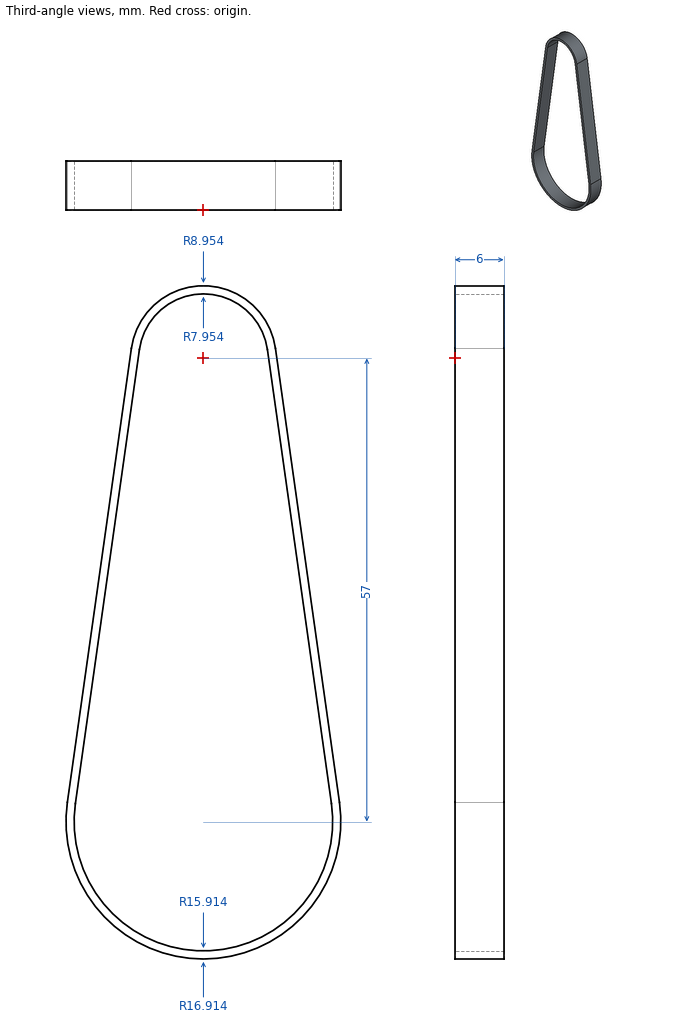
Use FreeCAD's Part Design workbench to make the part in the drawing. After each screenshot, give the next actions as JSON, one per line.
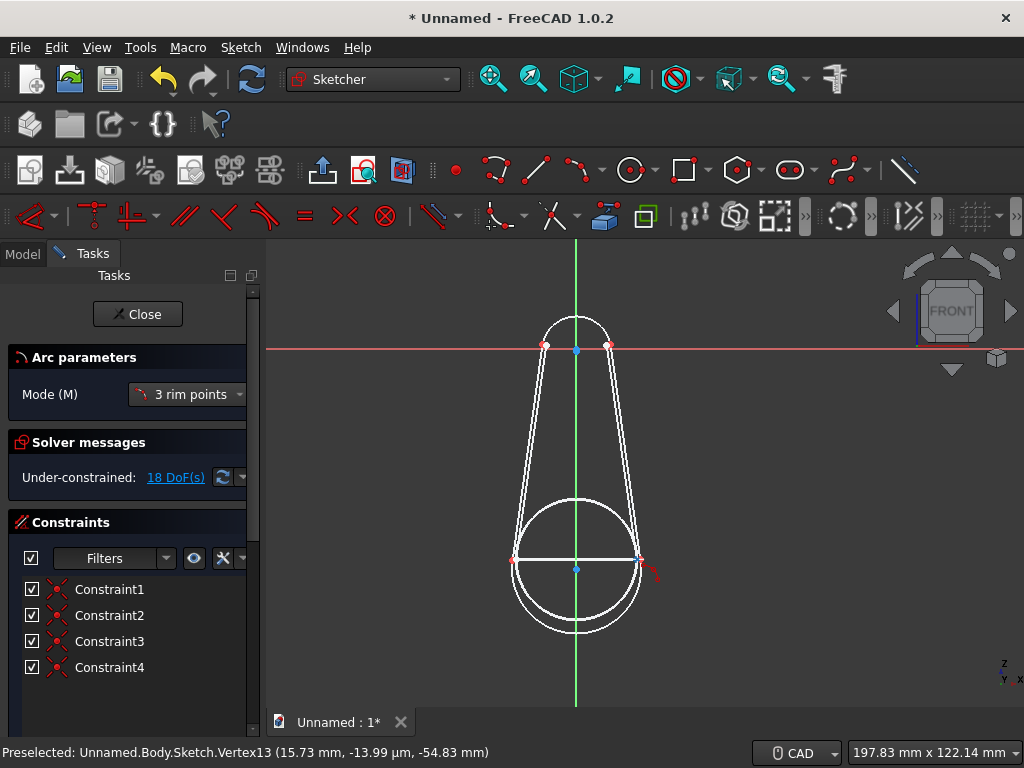
{"action": "scroll", "coordinate": [615, 615], "scroll_direction": "up", "scroll_amount": 8}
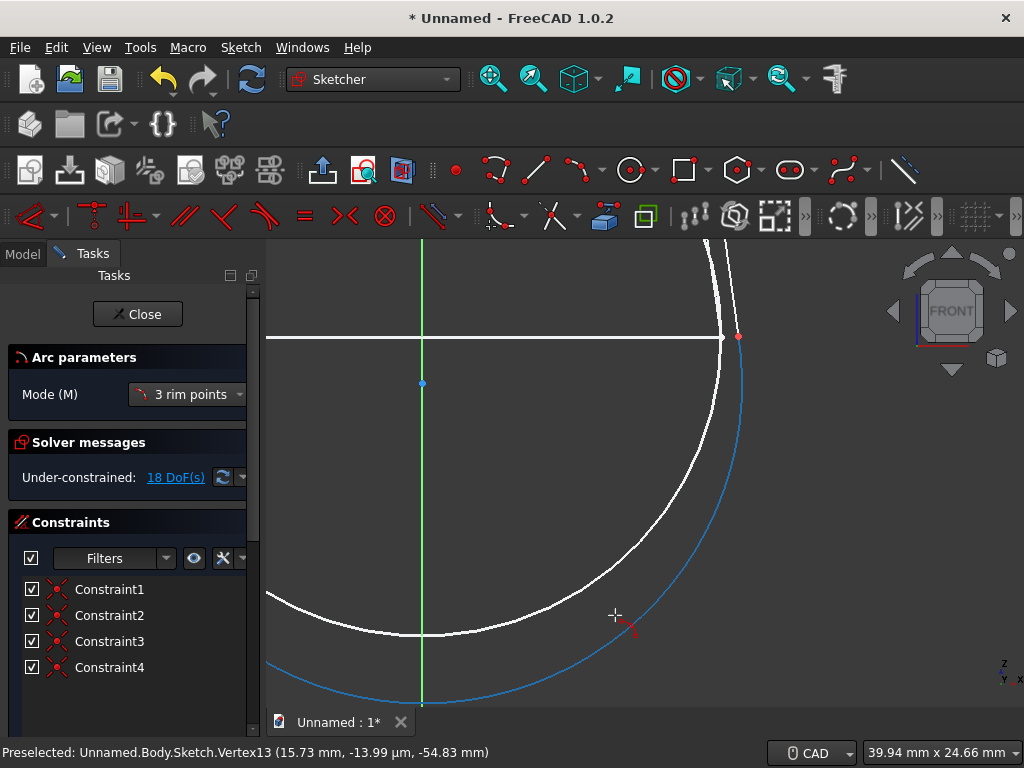
{"action": "left_click", "coordinate": [613, 612]}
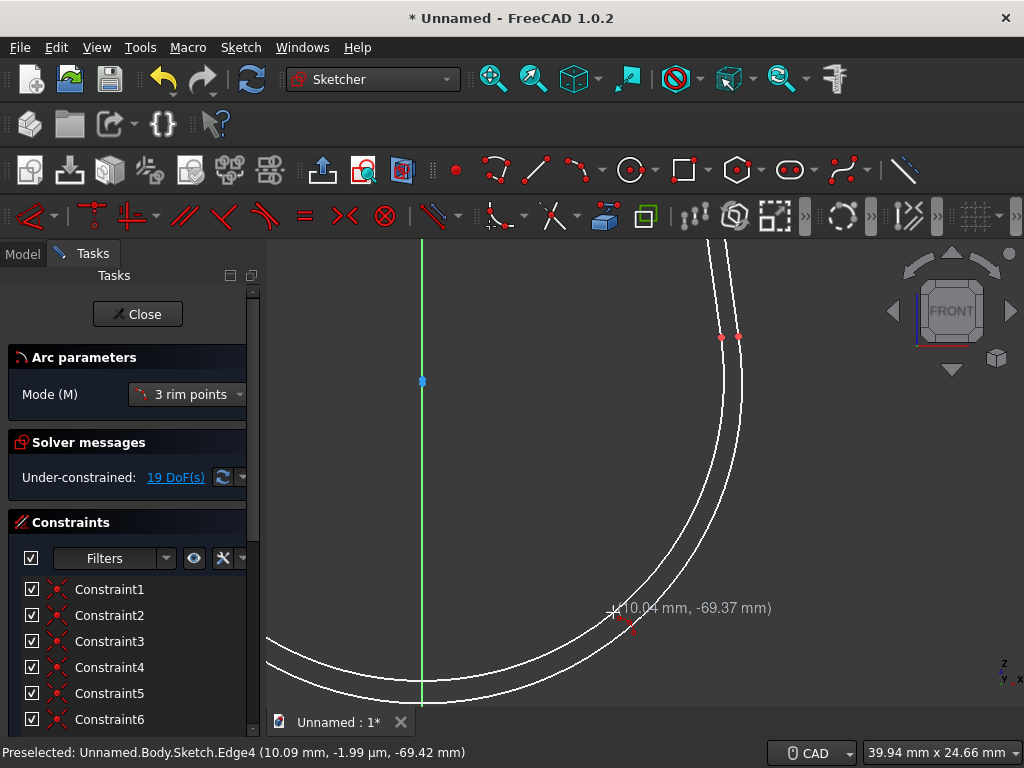
{"action": "scroll", "coordinate": [615, 615], "scroll_direction": "down", "scroll_amount": 8}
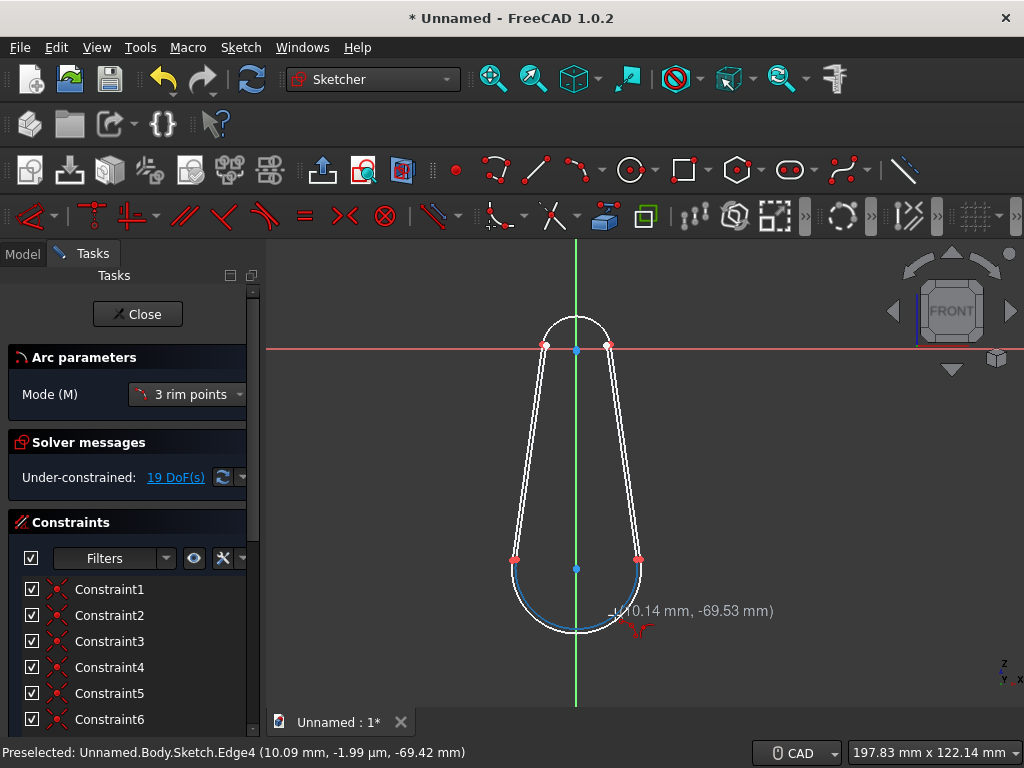
{"action": "scroll", "coordinate": [607, 345], "scroll_direction": "up", "scroll_amount": 8}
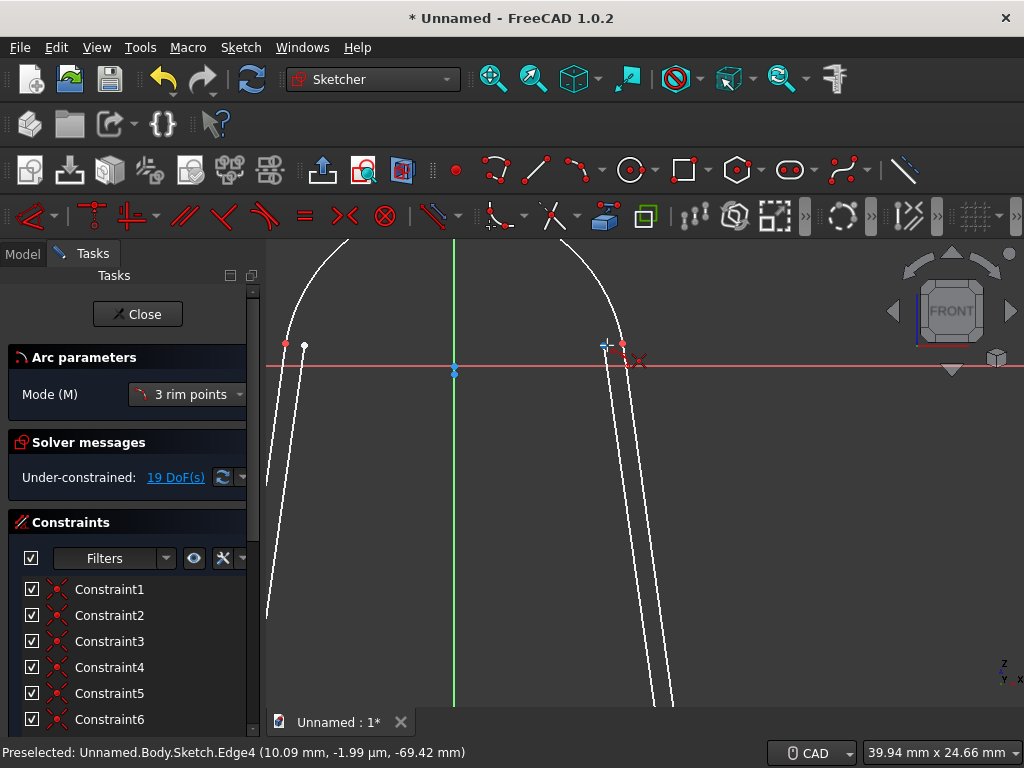
{"action": "left_click", "coordinate": [604, 346]}
{"action": "left_click", "coordinate": [305, 346]}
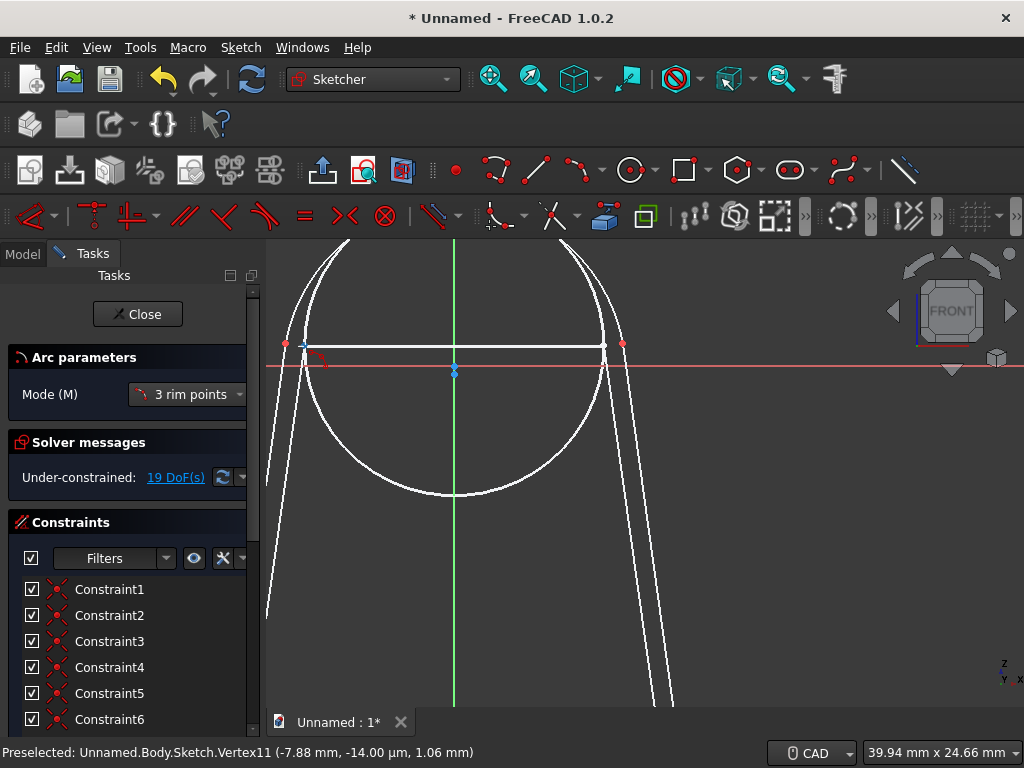
{"action": "scroll", "coordinate": [607, 344], "scroll_direction": "down", "scroll_amount": 8}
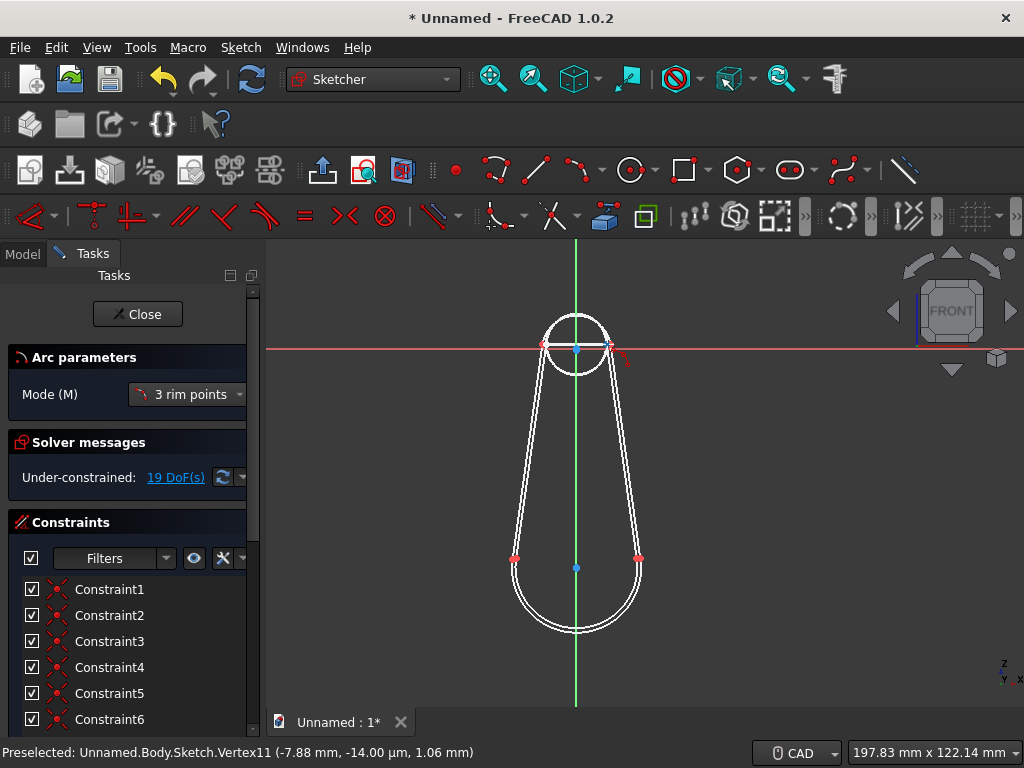
{"action": "scroll", "coordinate": [585, 319], "scroll_direction": "up", "scroll_amount": 8}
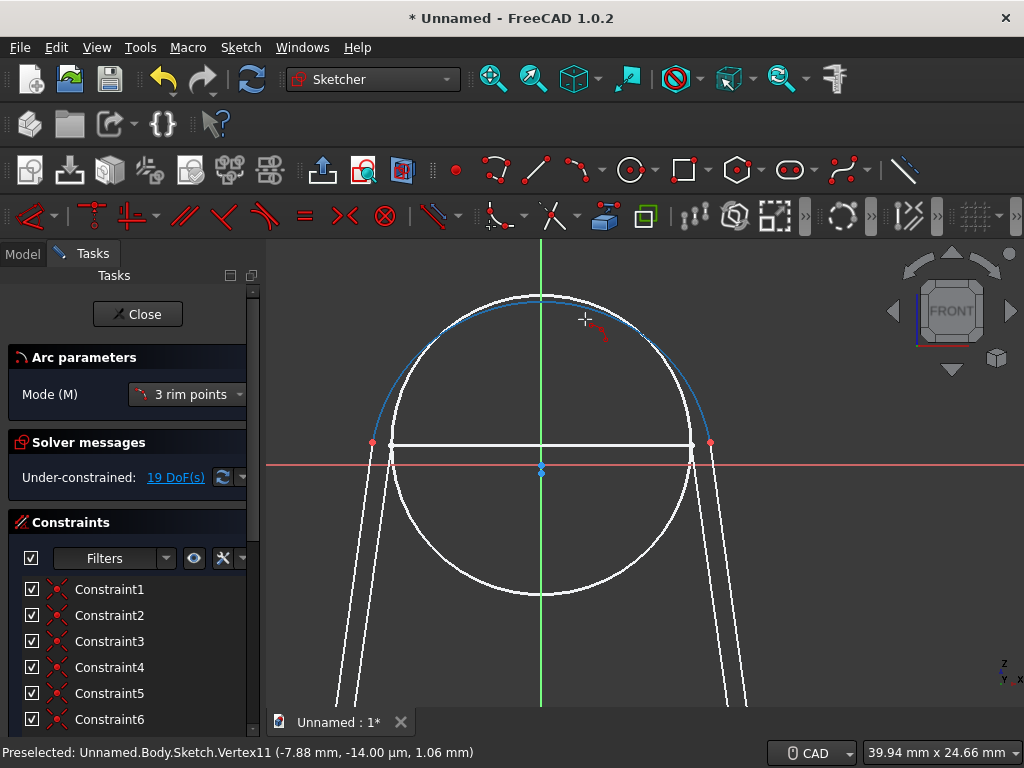
{"action": "left_click", "coordinate": [584, 320]}
{"action": "key", "text": "Escape"}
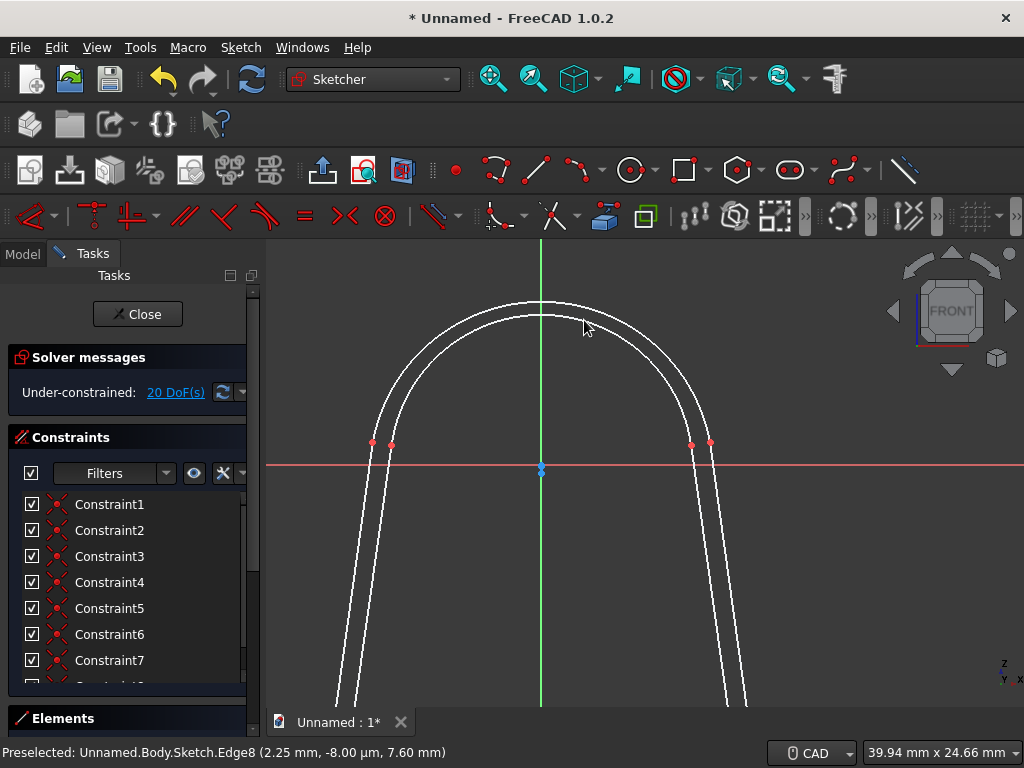
{"action": "left_click", "coordinate": [343, 656]}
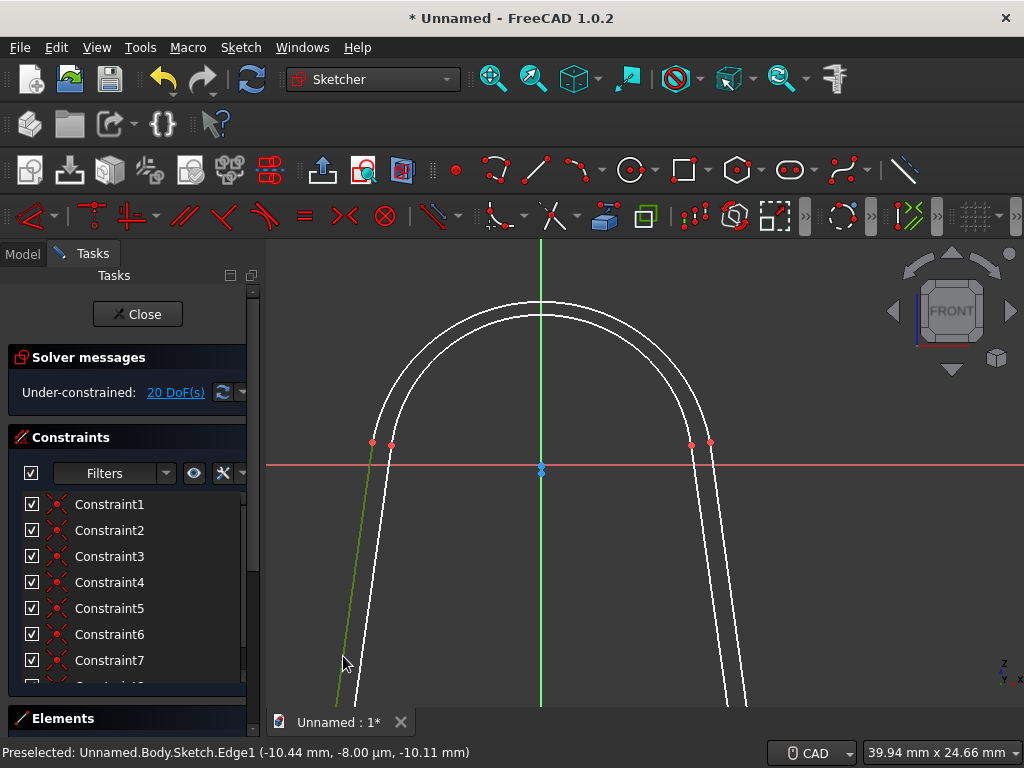
{"action": "left_click", "coordinate": [632, 328]}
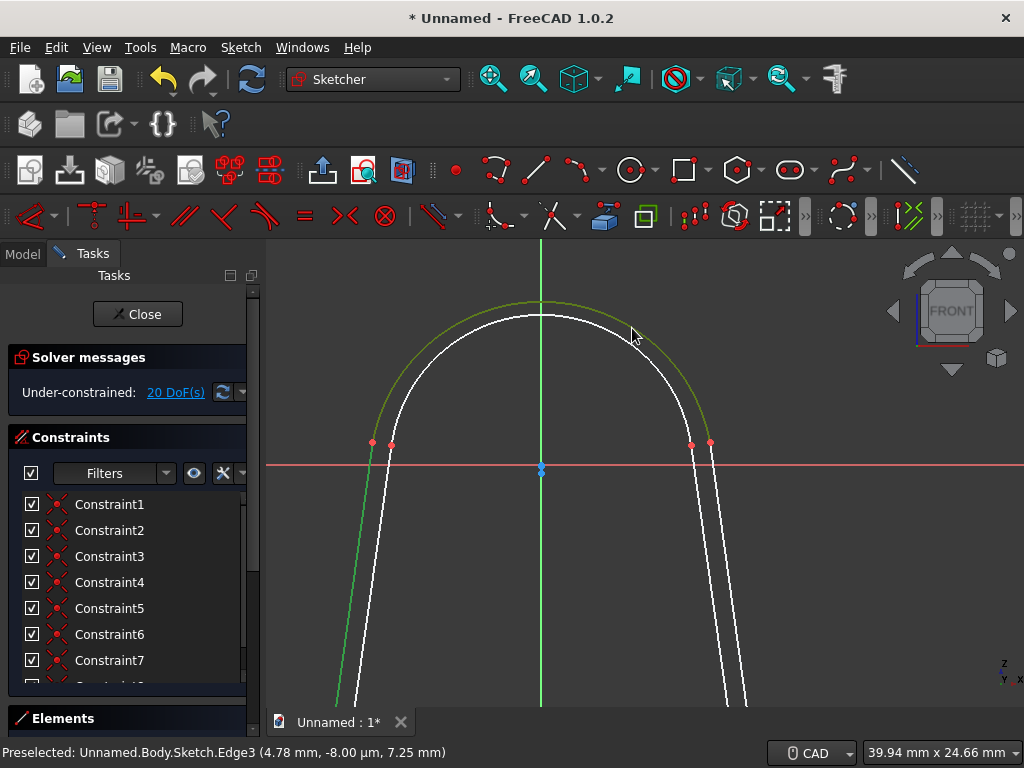
{"action": "left_click", "coordinate": [266, 216]}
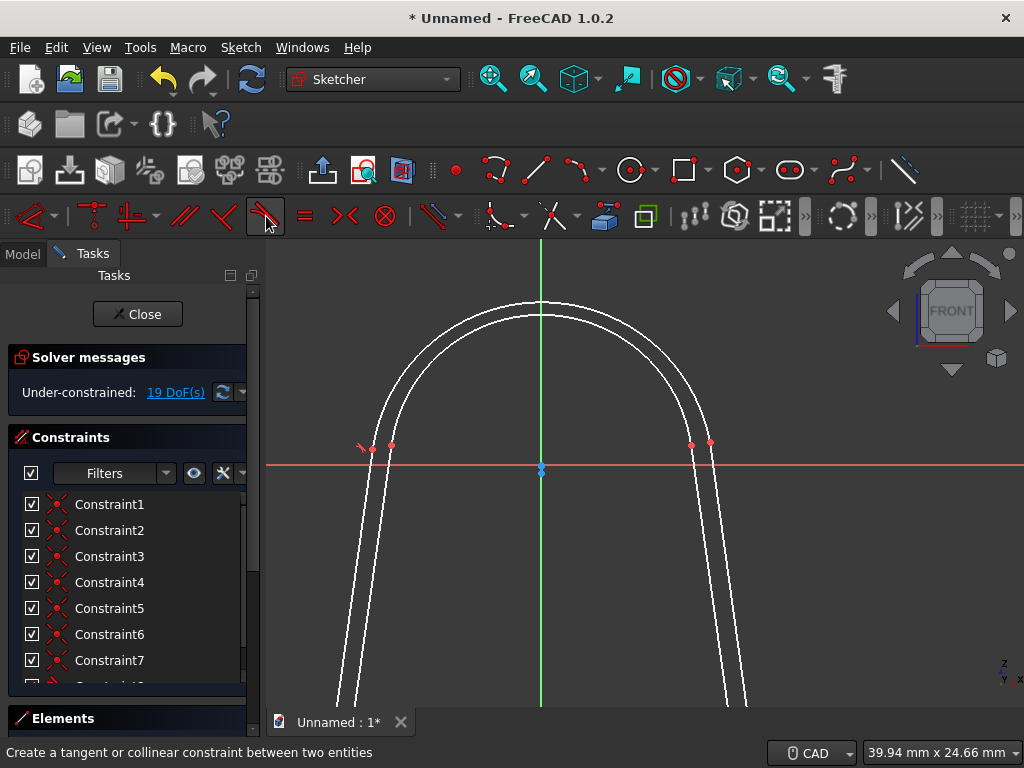
{"action": "left_click", "coordinate": [343, 661]}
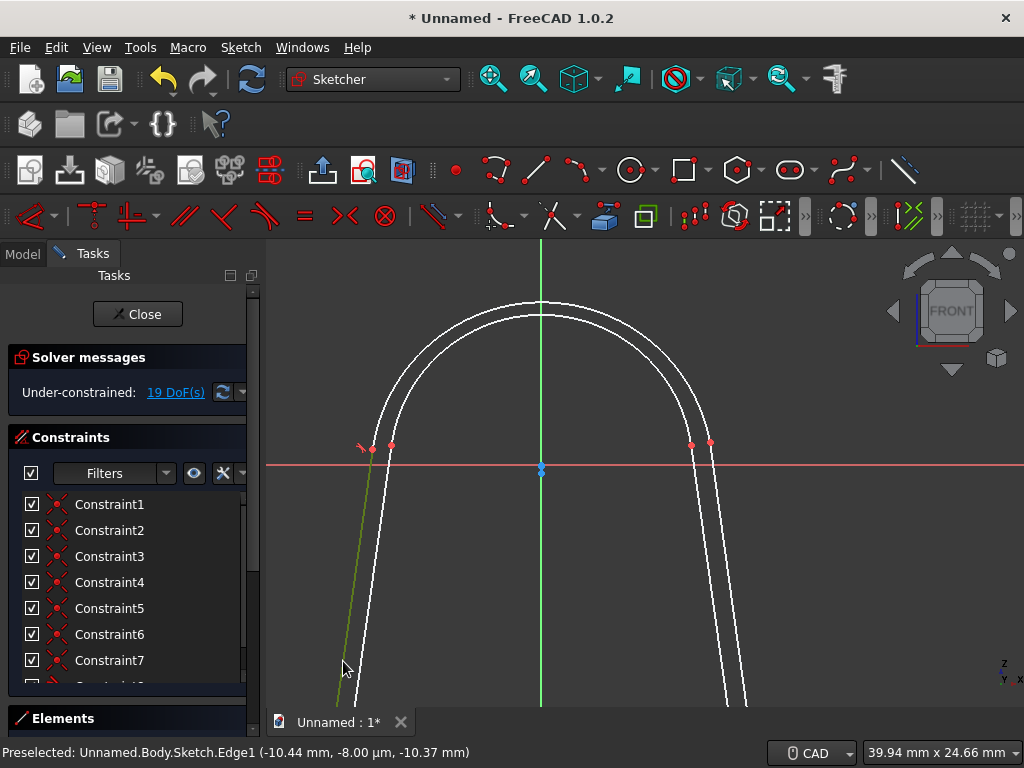
{"action": "scroll", "coordinate": [585, 319], "scroll_direction": "down", "scroll_amount": 8}